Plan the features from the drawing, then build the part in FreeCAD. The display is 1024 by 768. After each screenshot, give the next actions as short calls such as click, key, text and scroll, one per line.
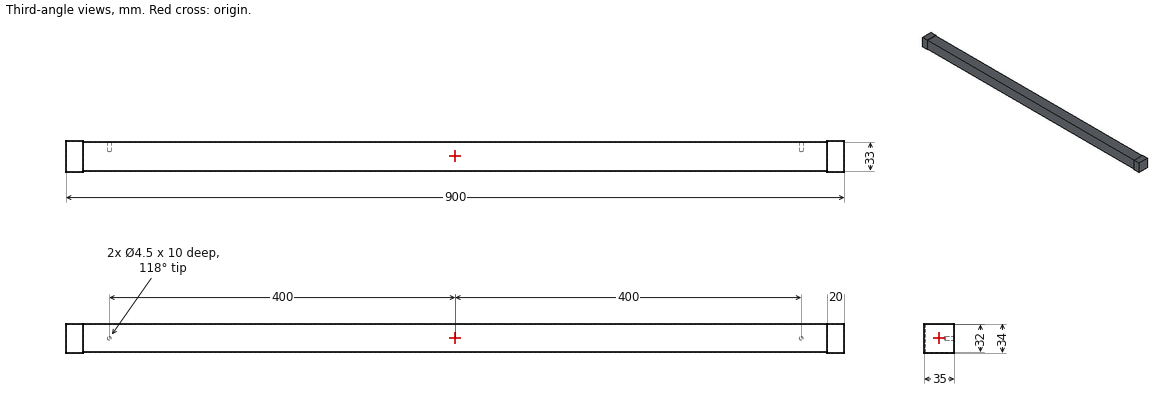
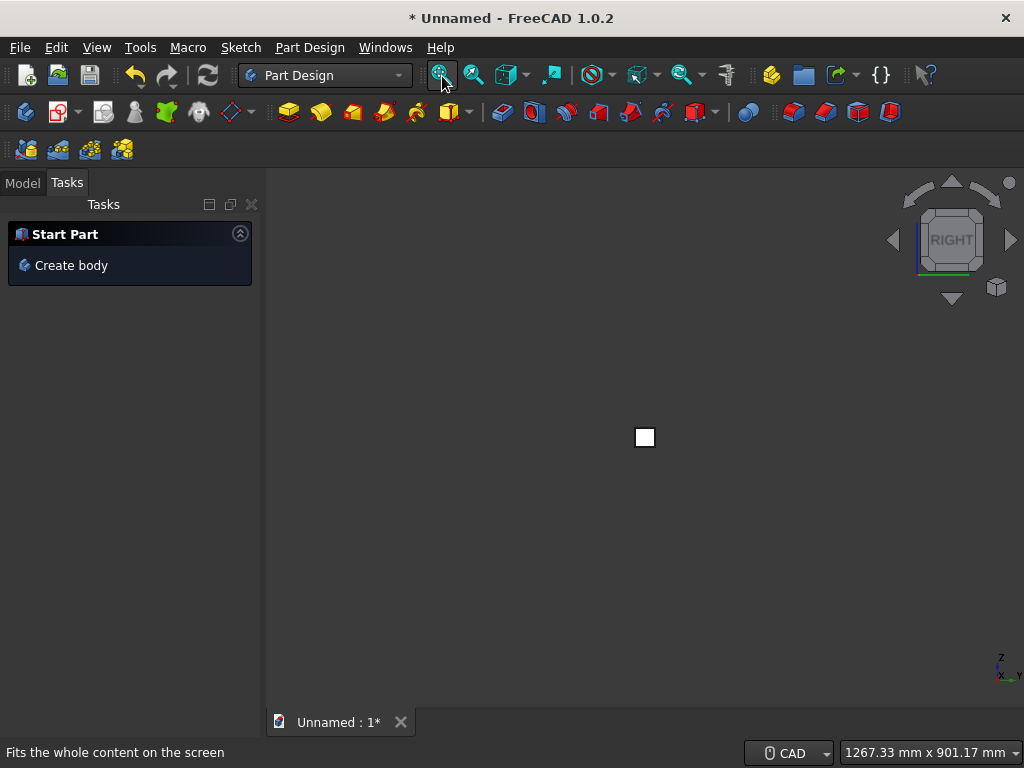
click(645, 436)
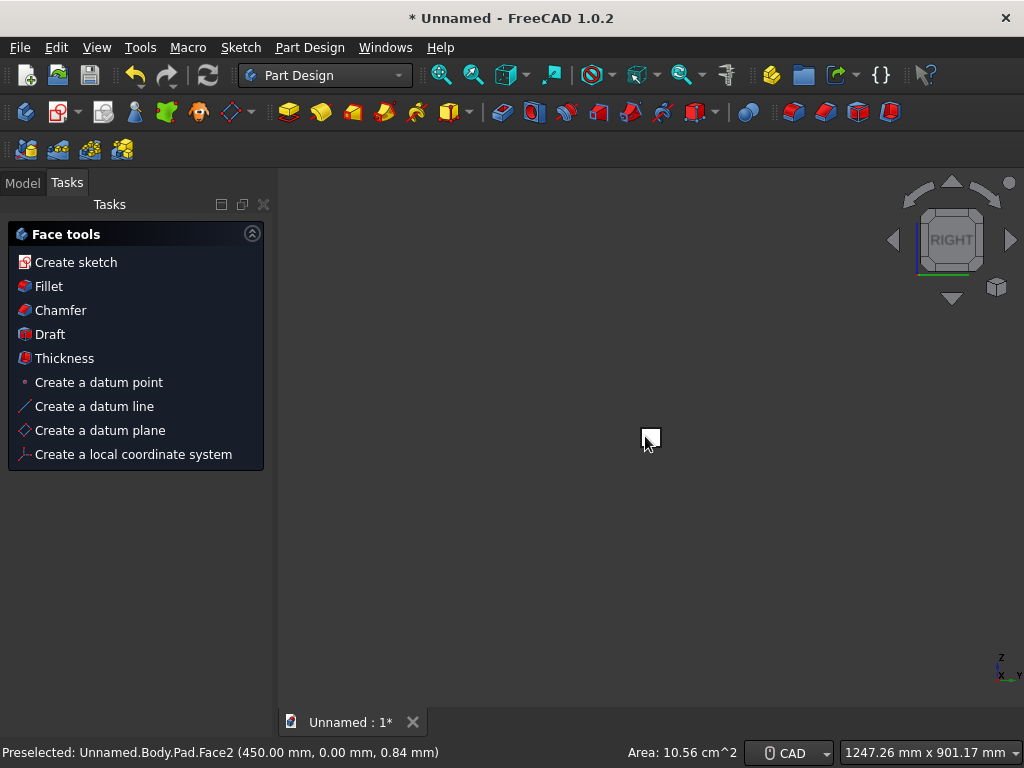
click(58, 112)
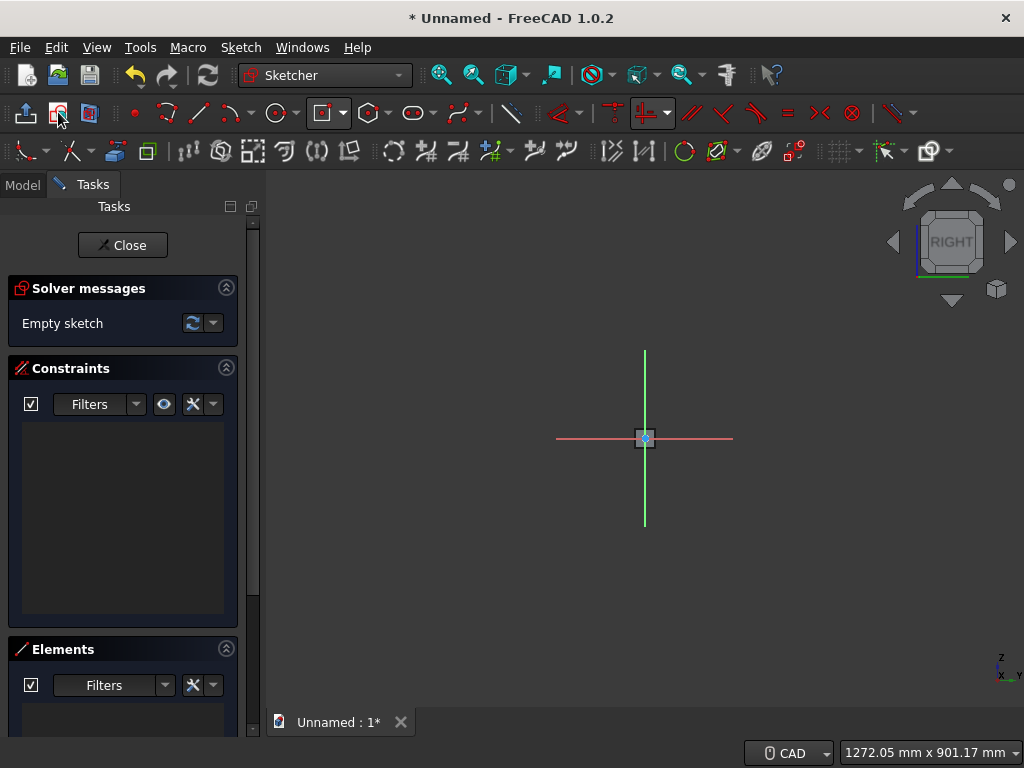
scroll(649, 438, up, 14)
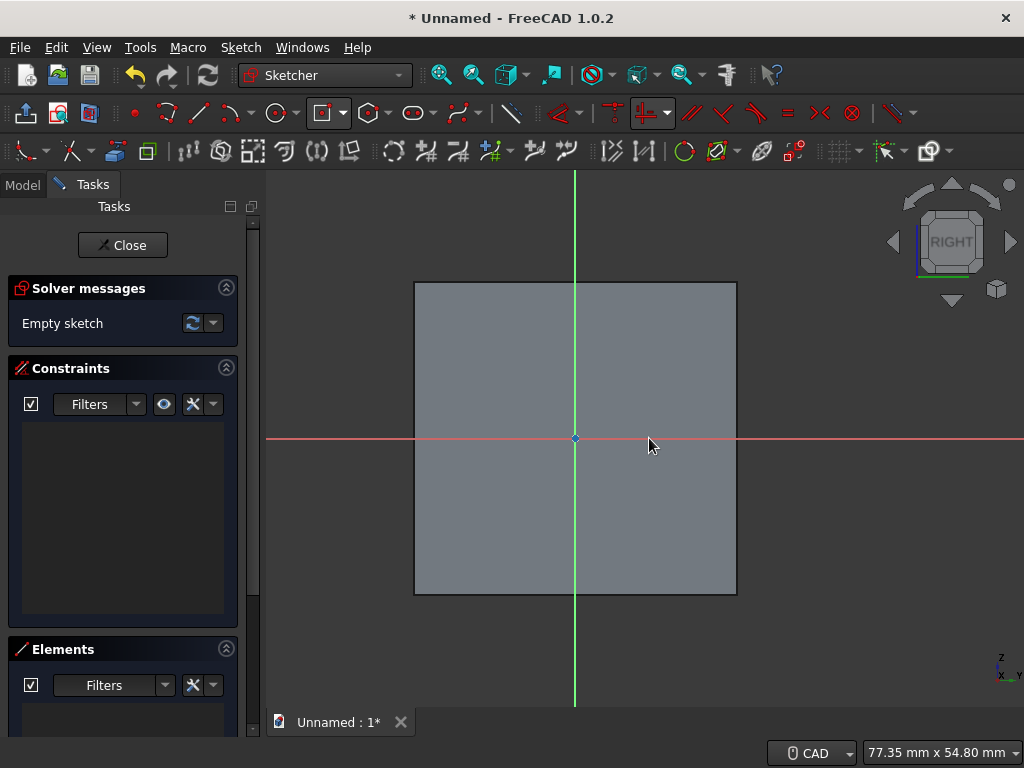
key(g)
key(v)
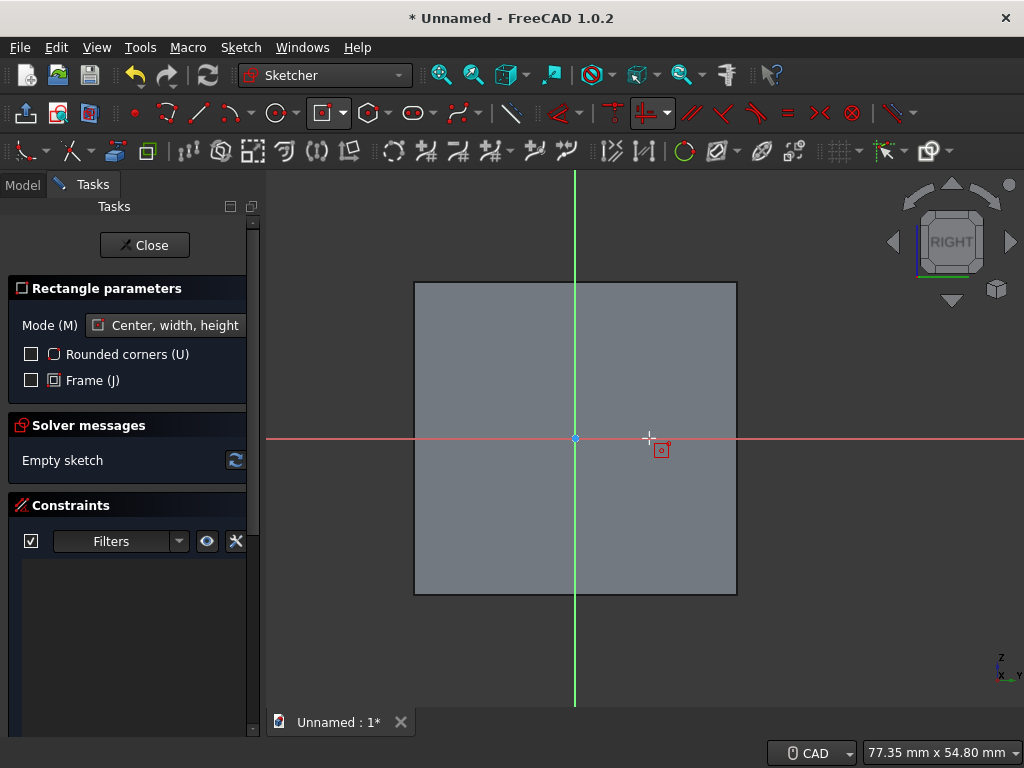
click(575, 438)
click(747, 272)
key(Escape)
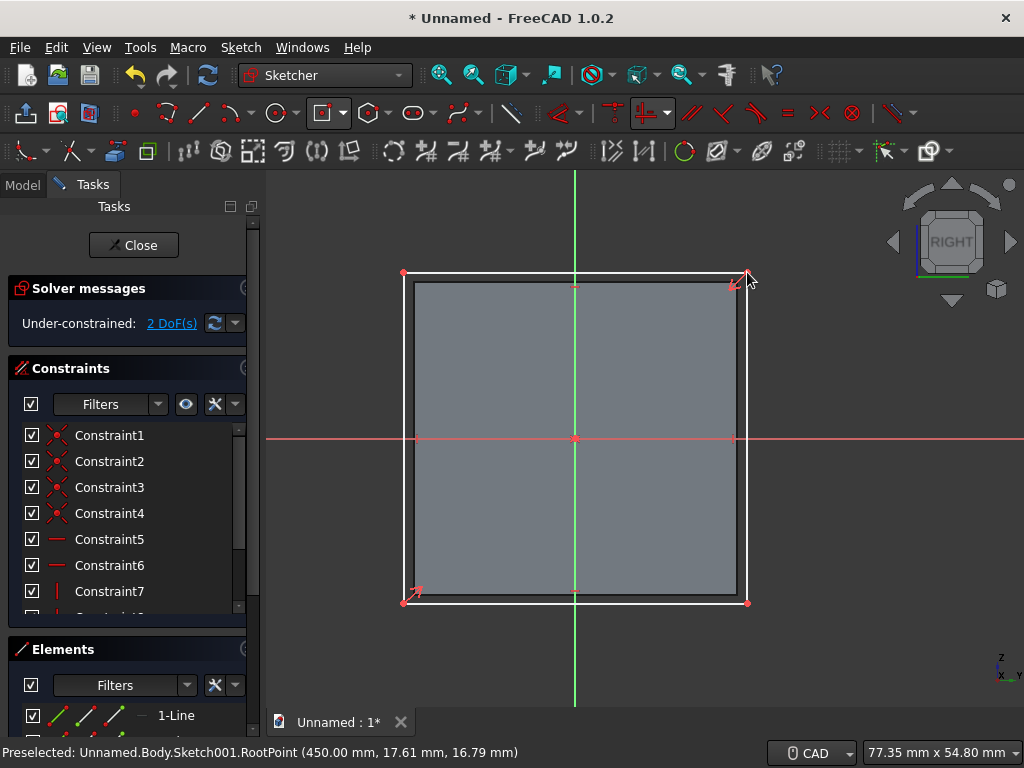
click(507, 604)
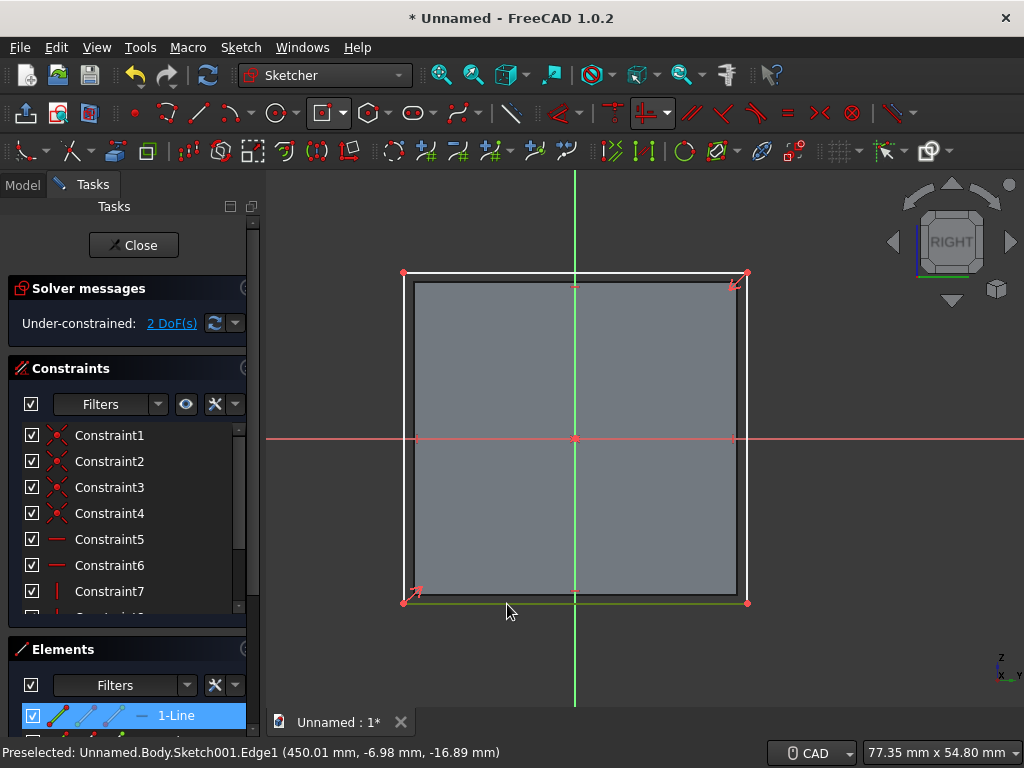
key(l)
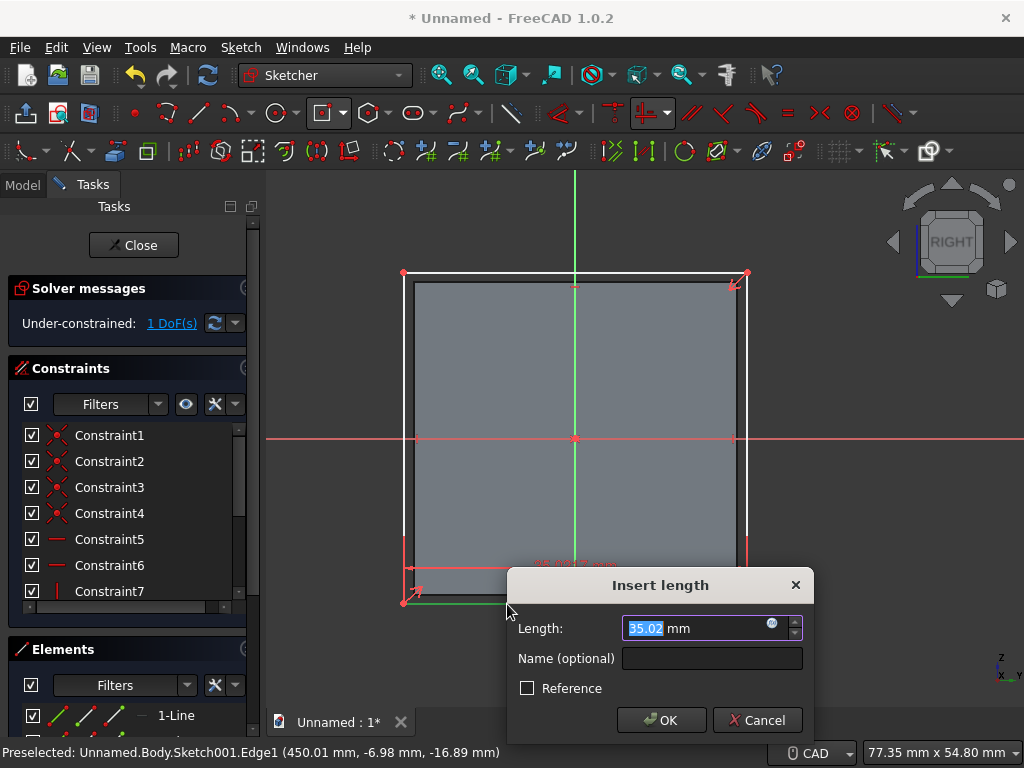
text(35)
key(Return)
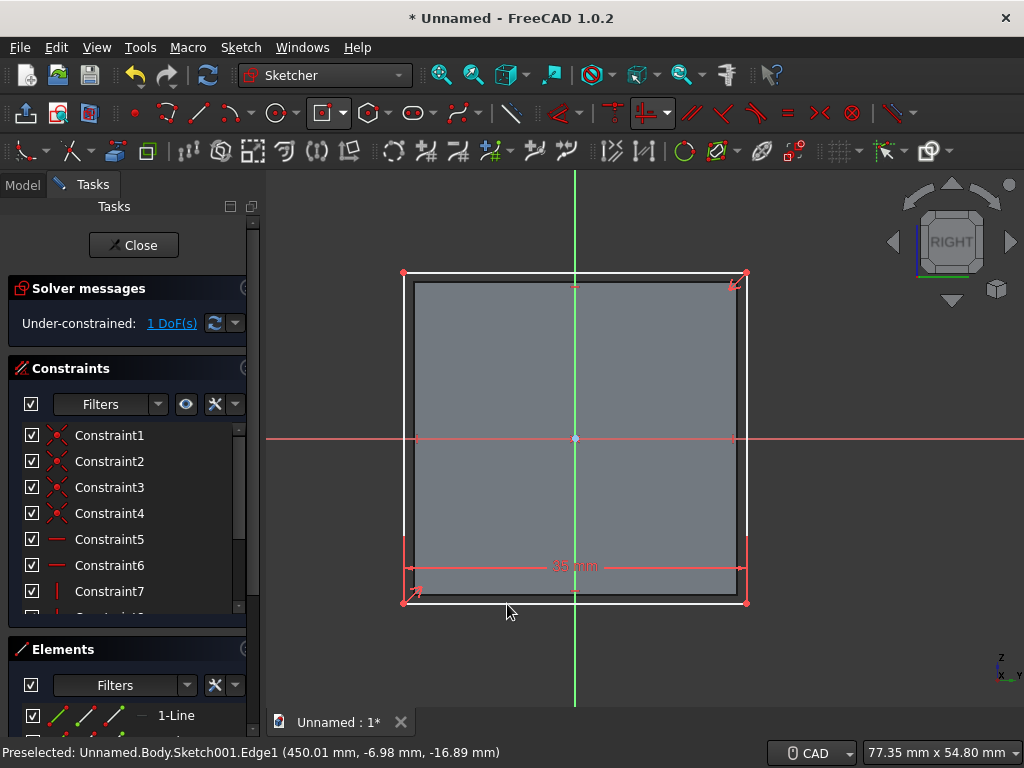
click(747, 505)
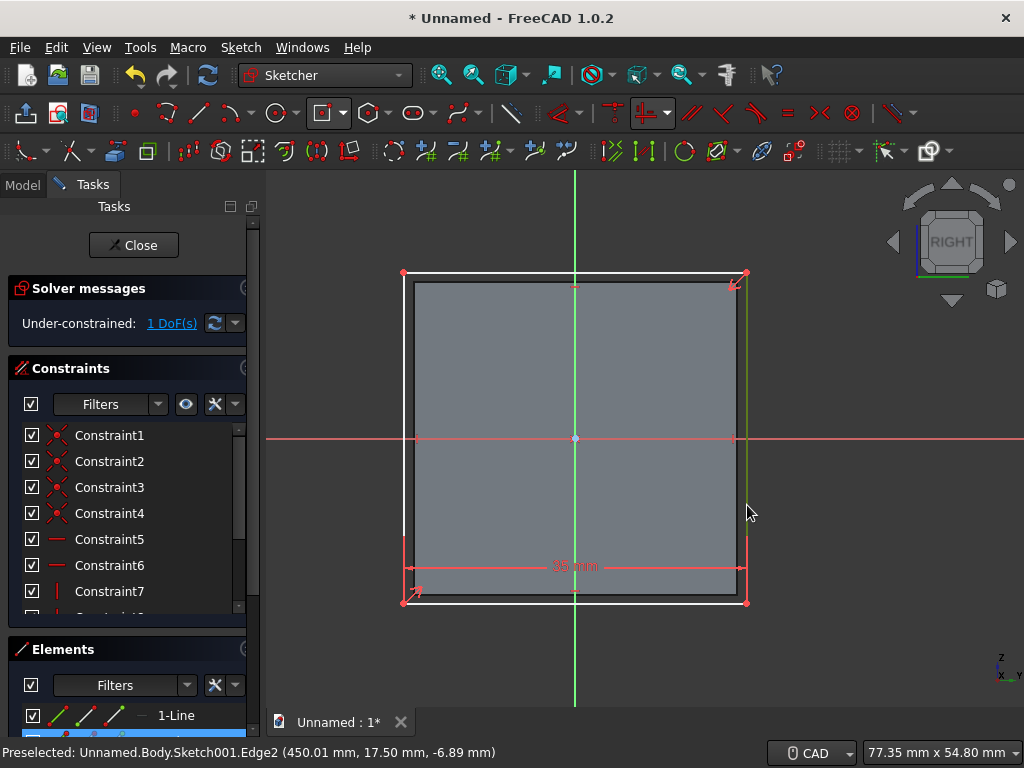
key(i)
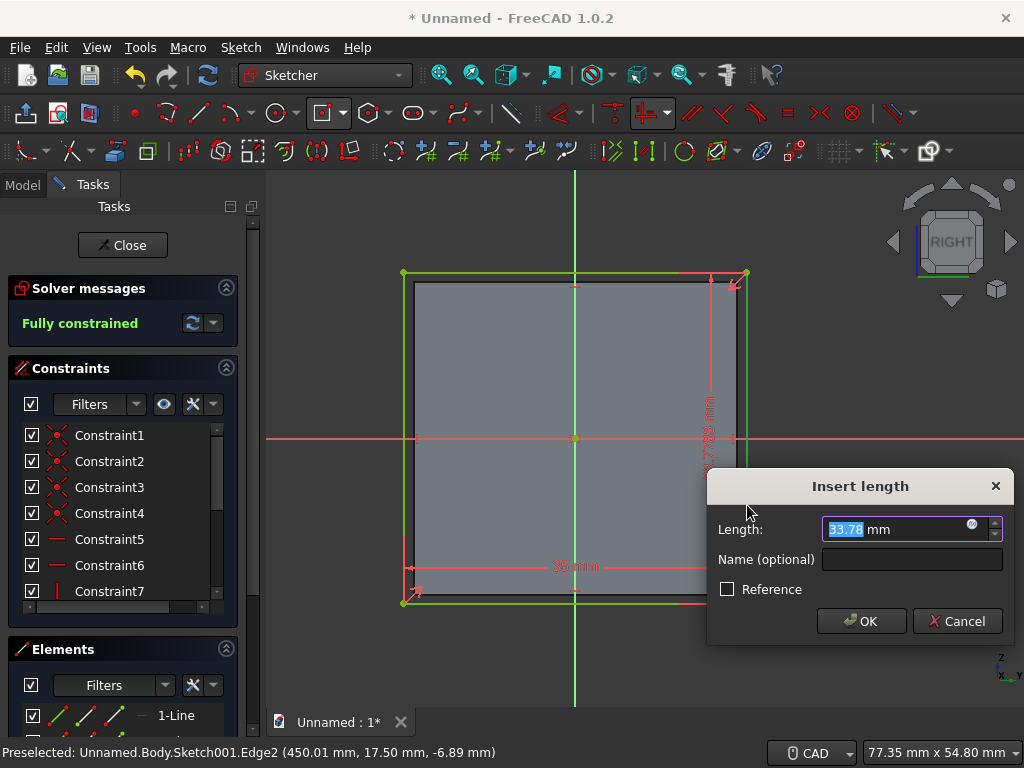
text(34)
key(Return)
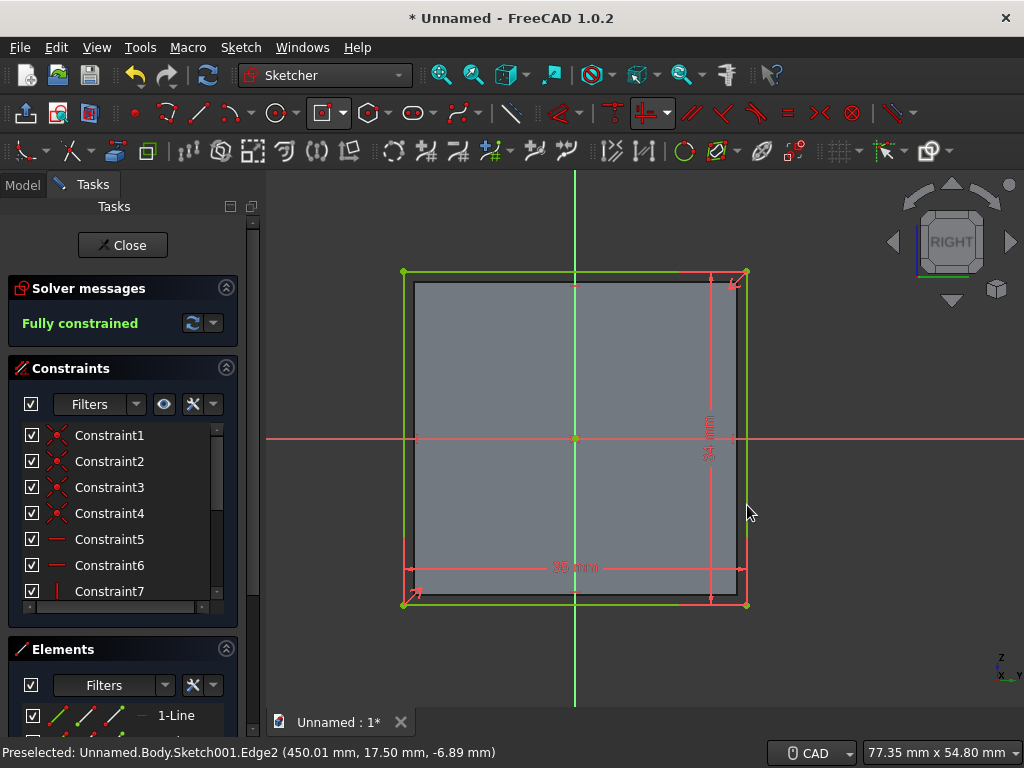
click(123, 245)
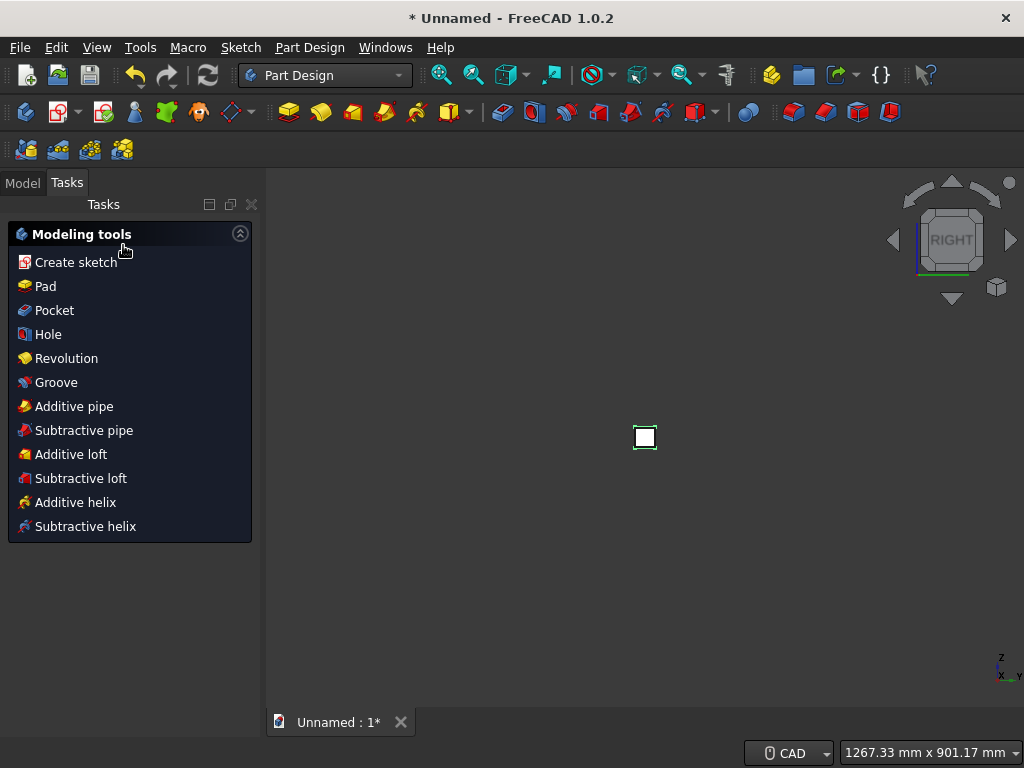
click(290, 112)